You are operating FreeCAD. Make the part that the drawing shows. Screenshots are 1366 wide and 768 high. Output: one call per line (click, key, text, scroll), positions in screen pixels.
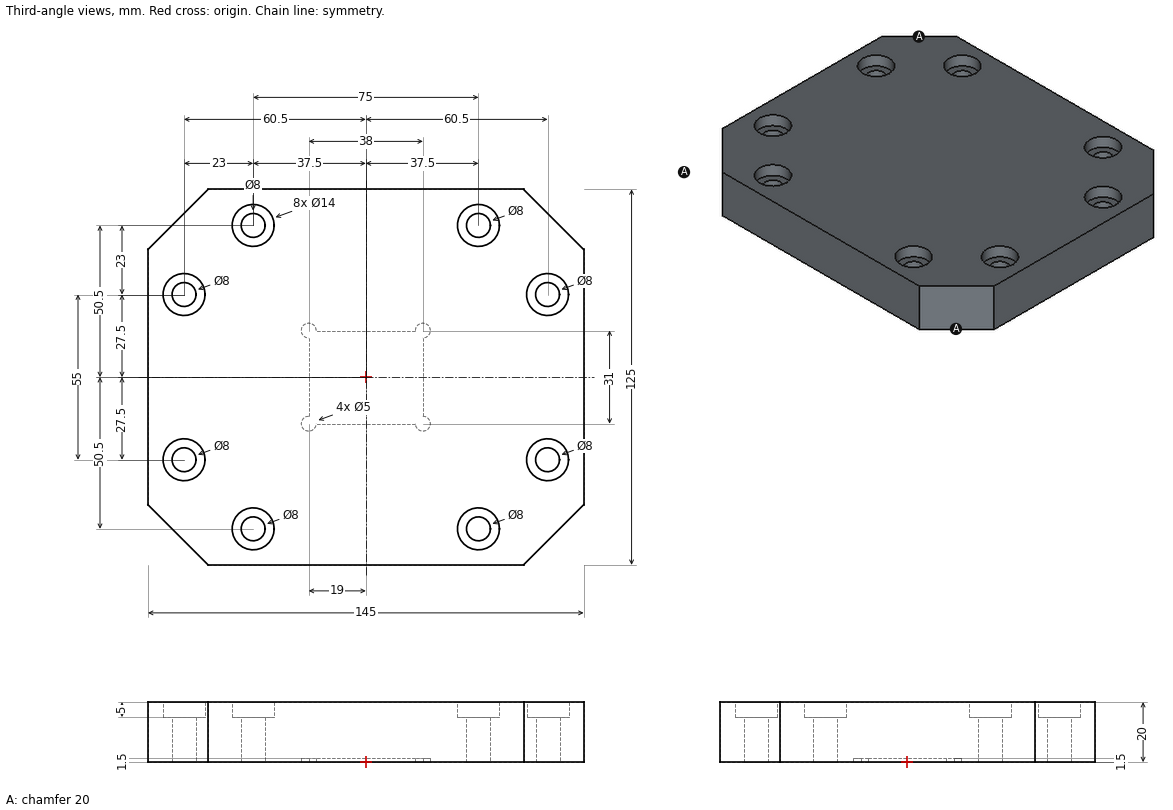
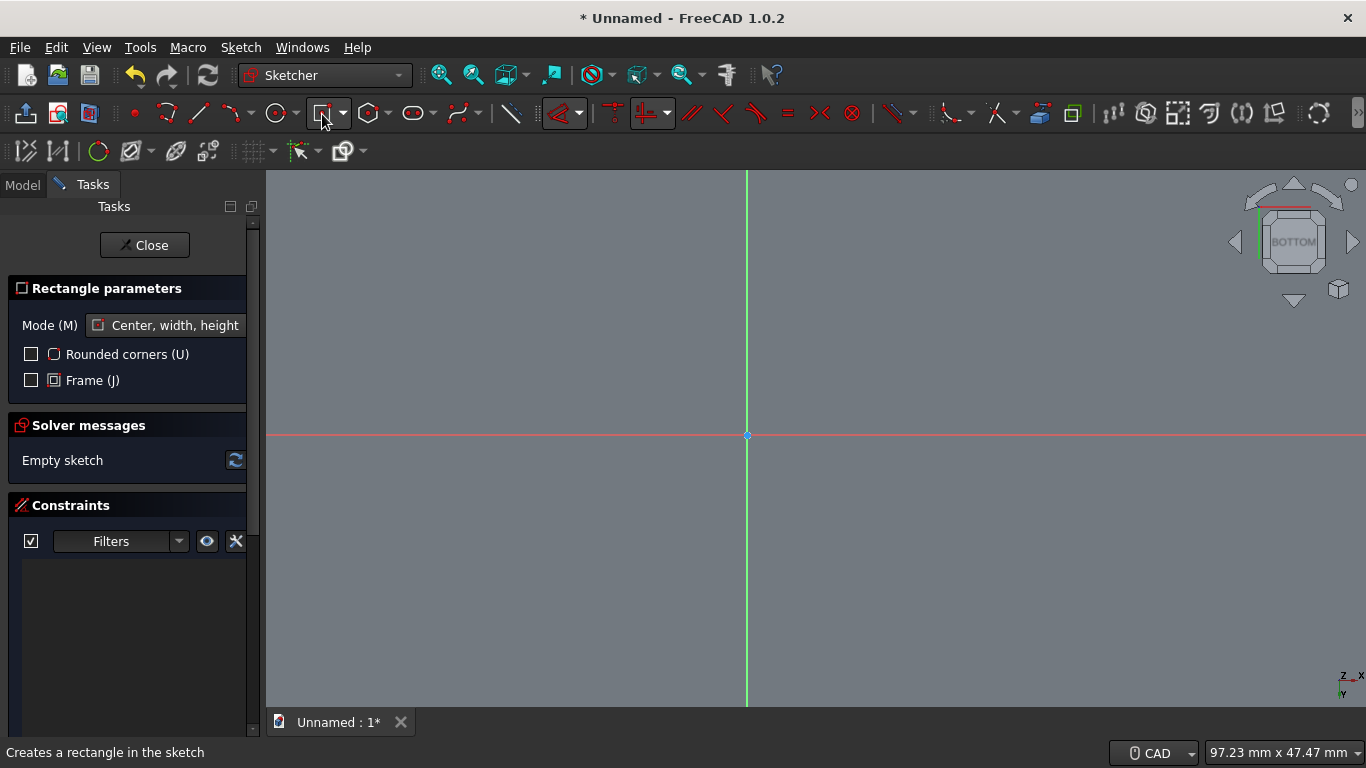
click(747, 435)
click(962, 260)
key(Escape)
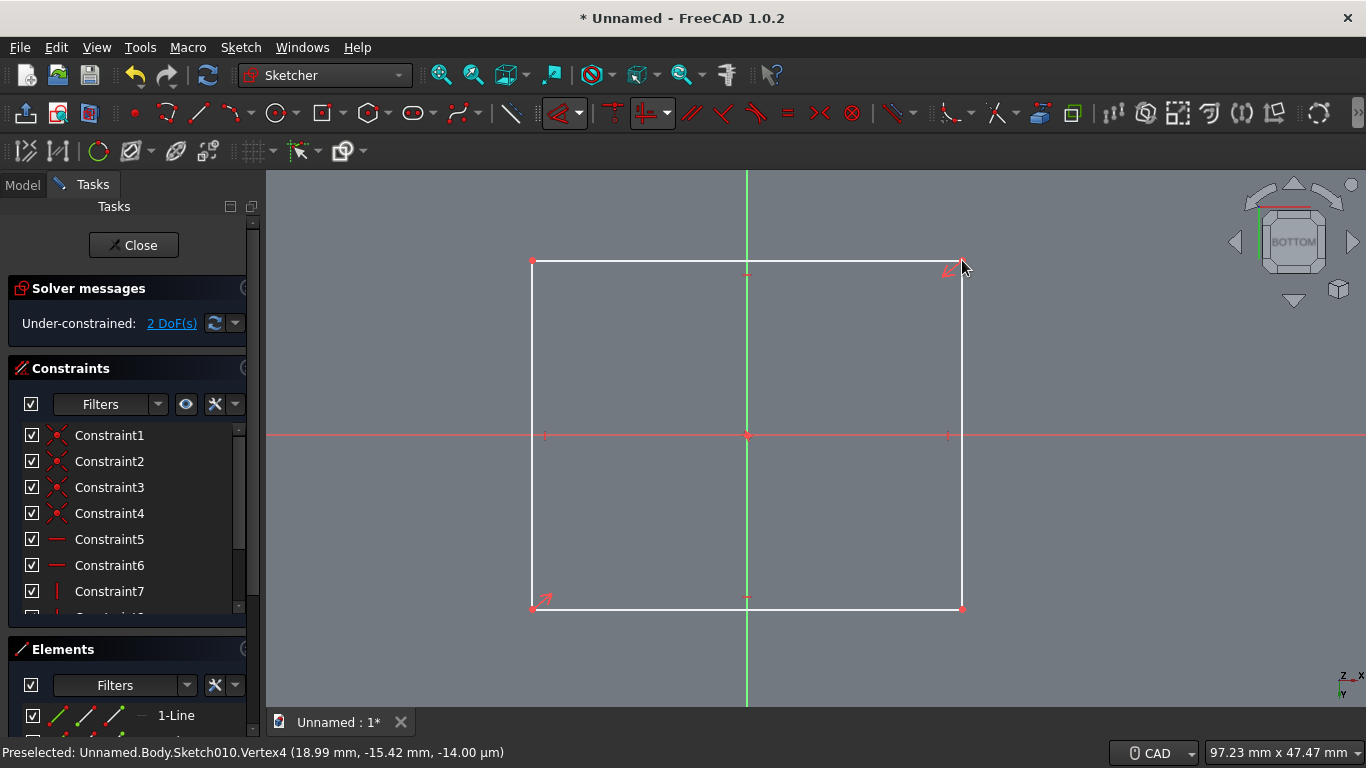
click(661, 610)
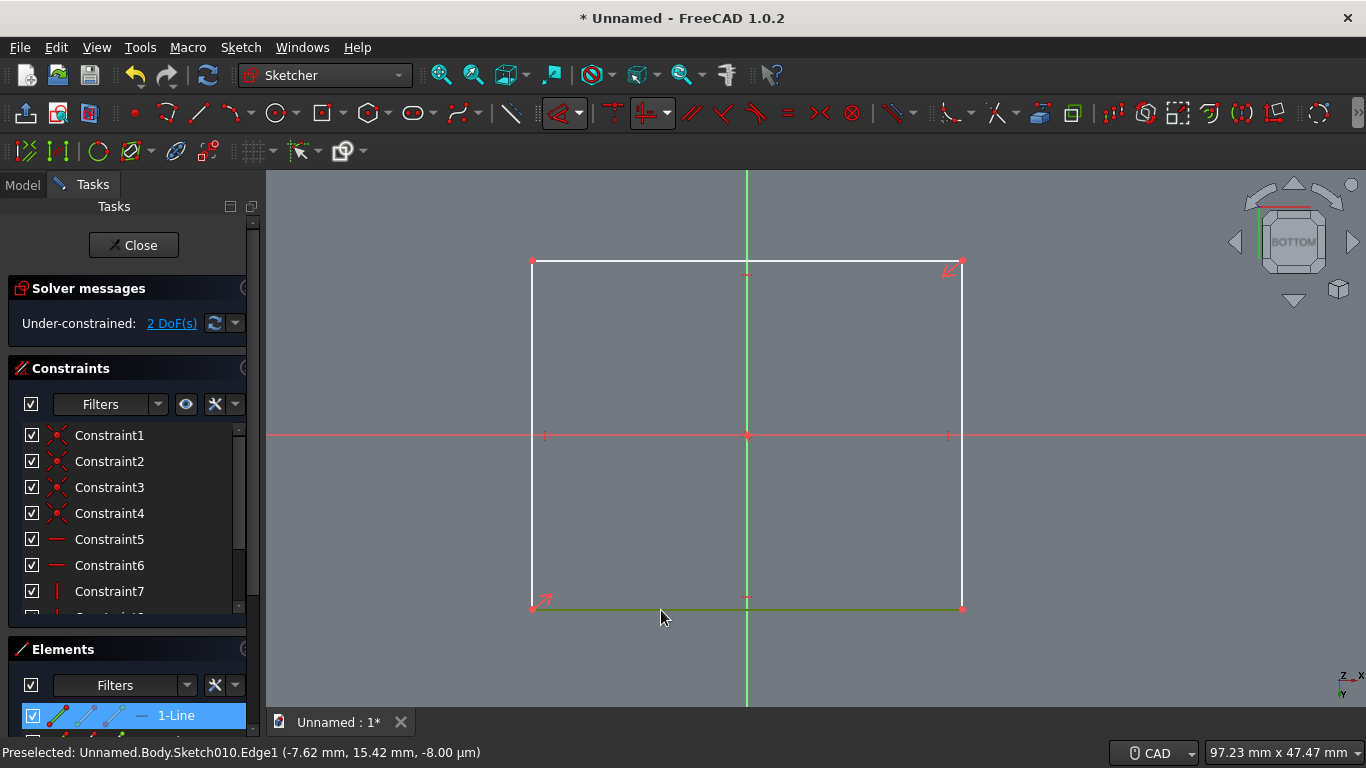
key(l)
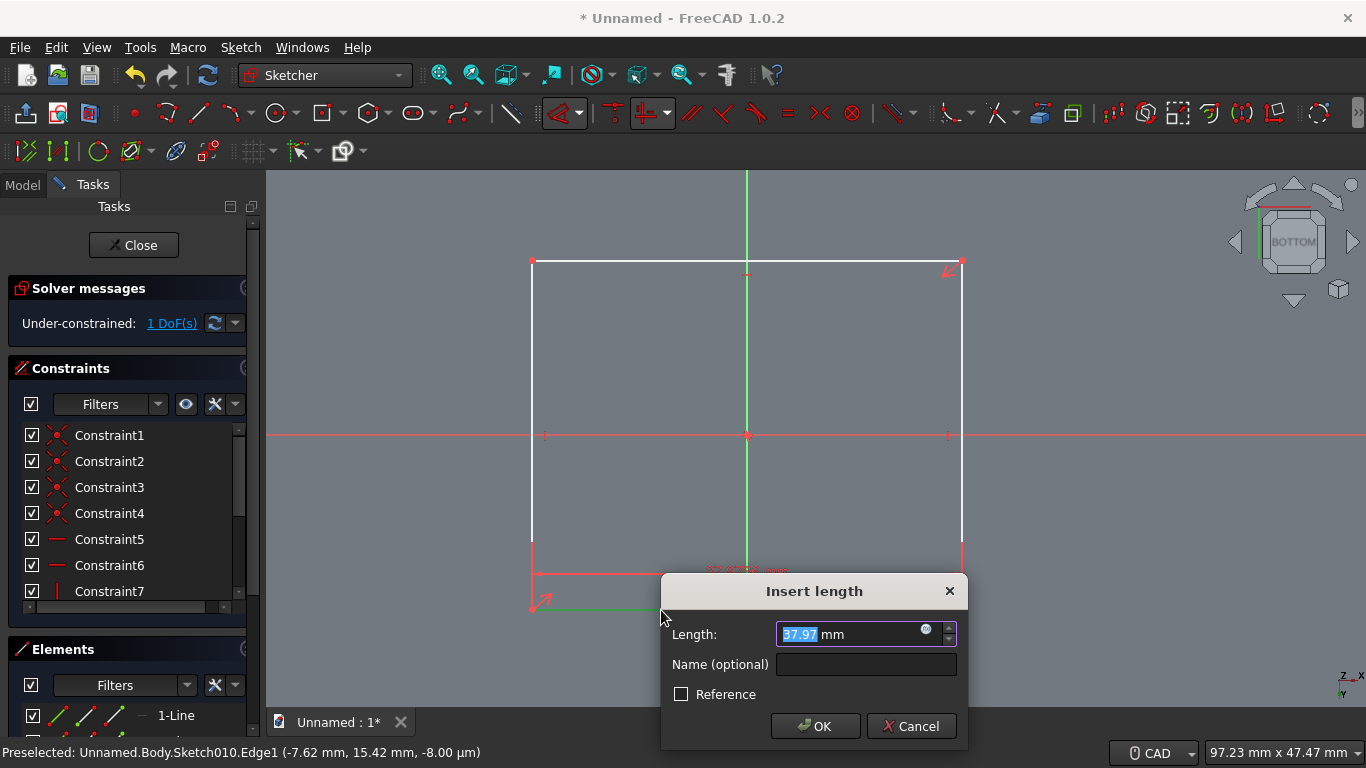
text(38)
key(Return)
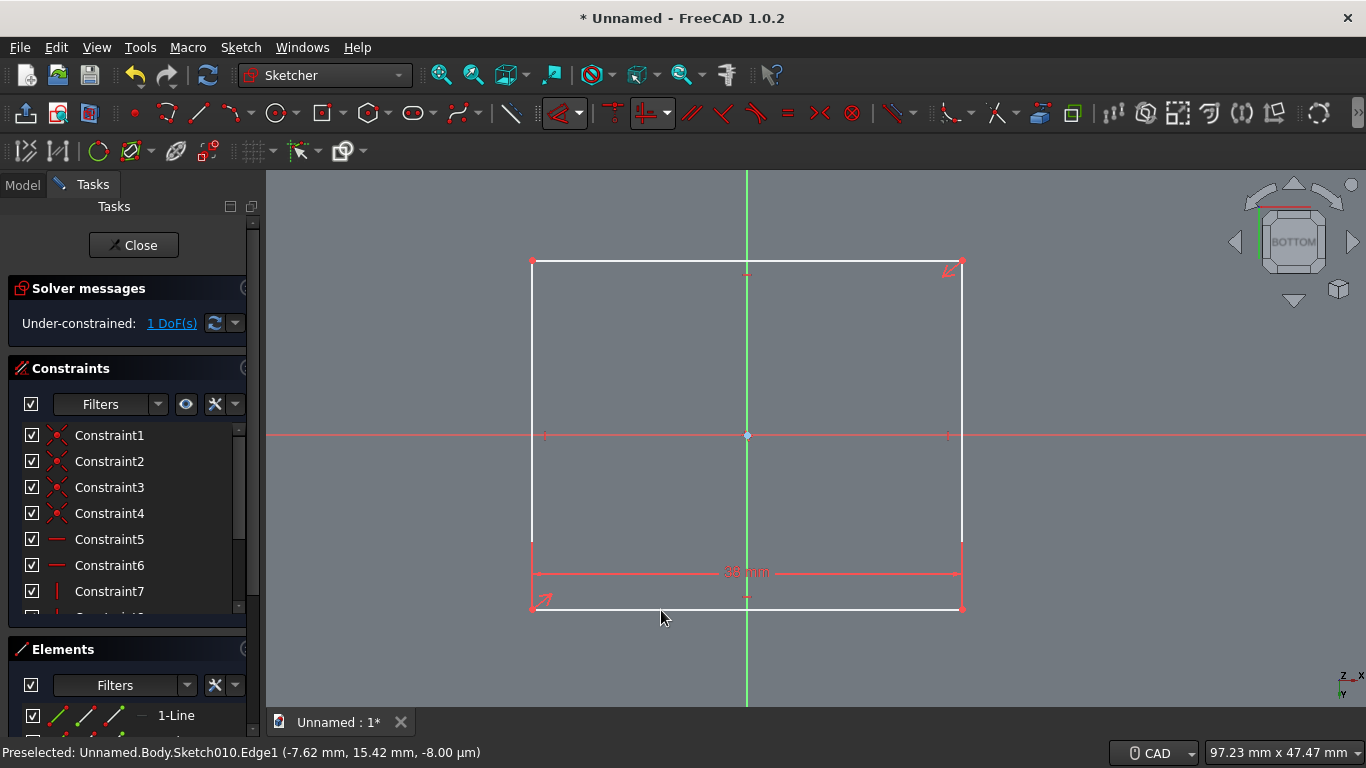
click(962, 505)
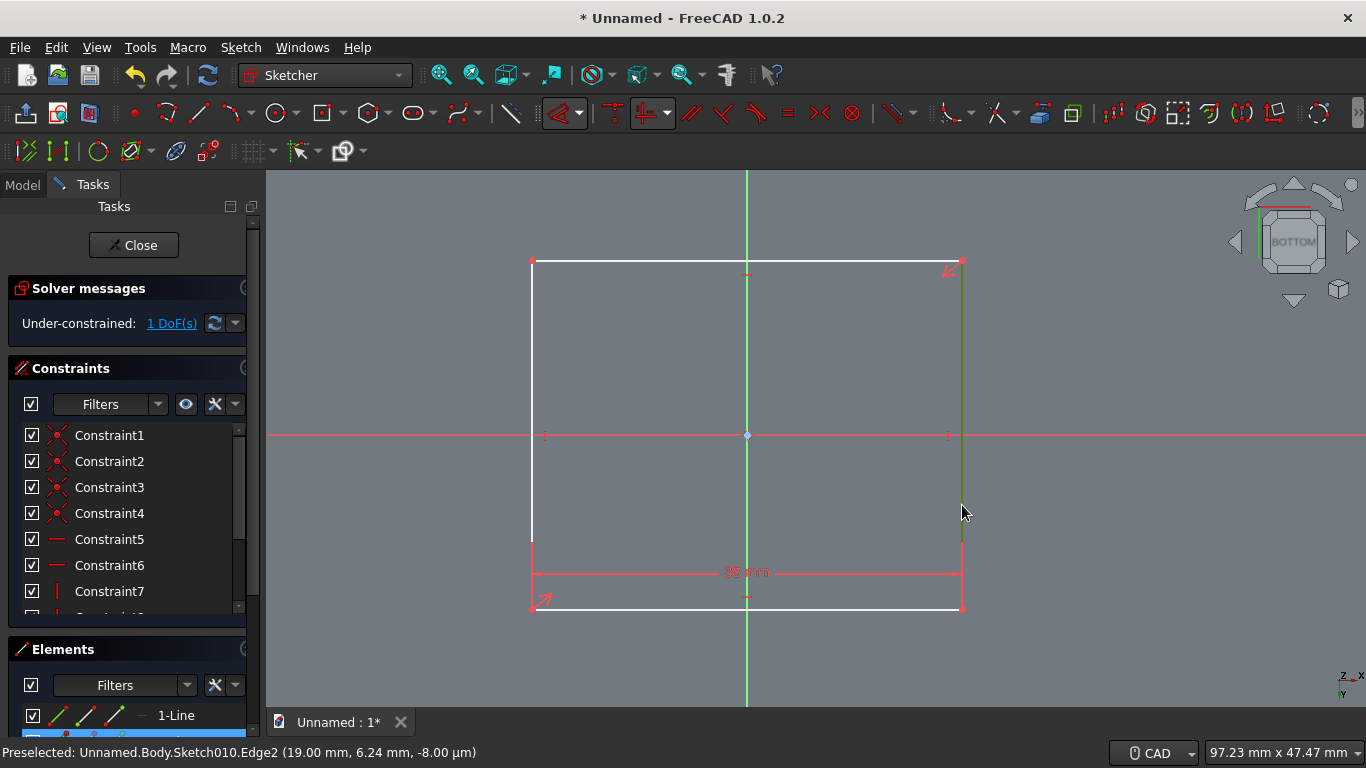
key(i)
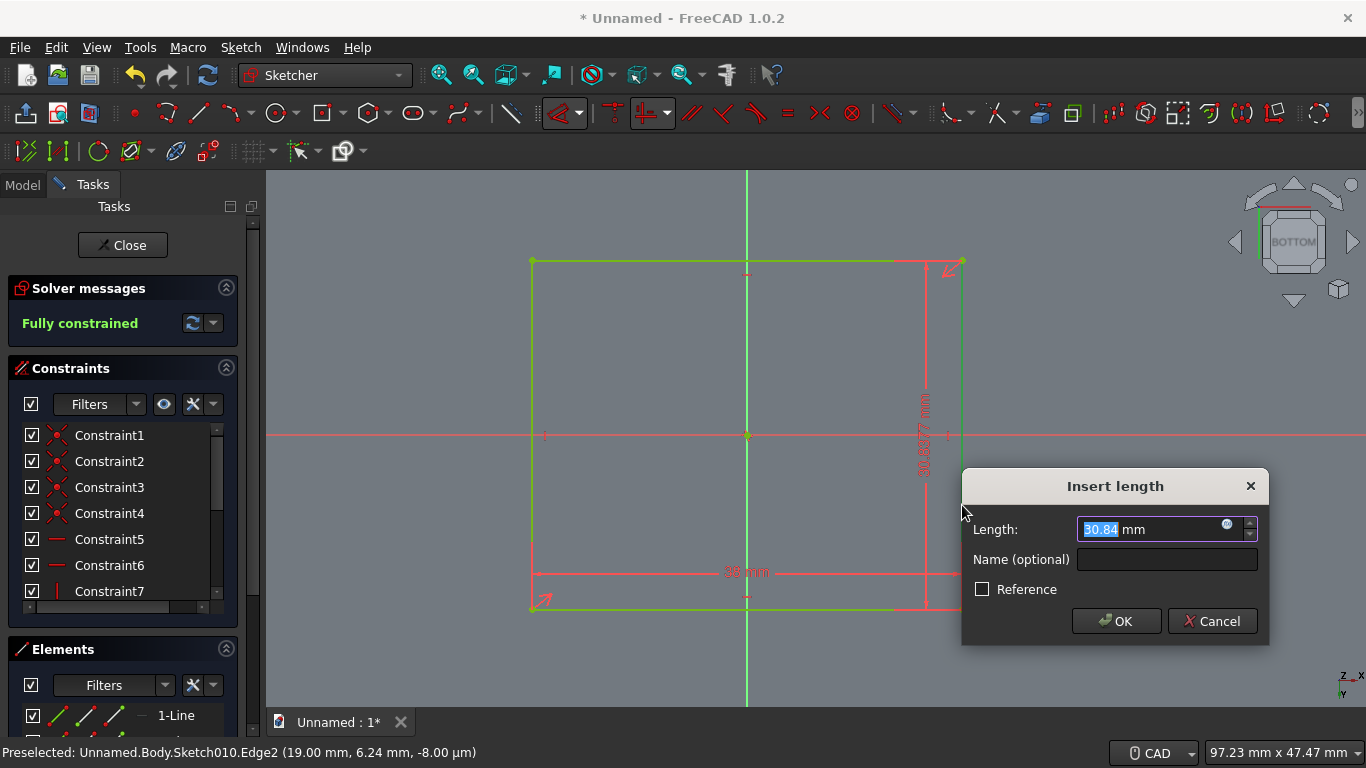
text(31)
key(Return)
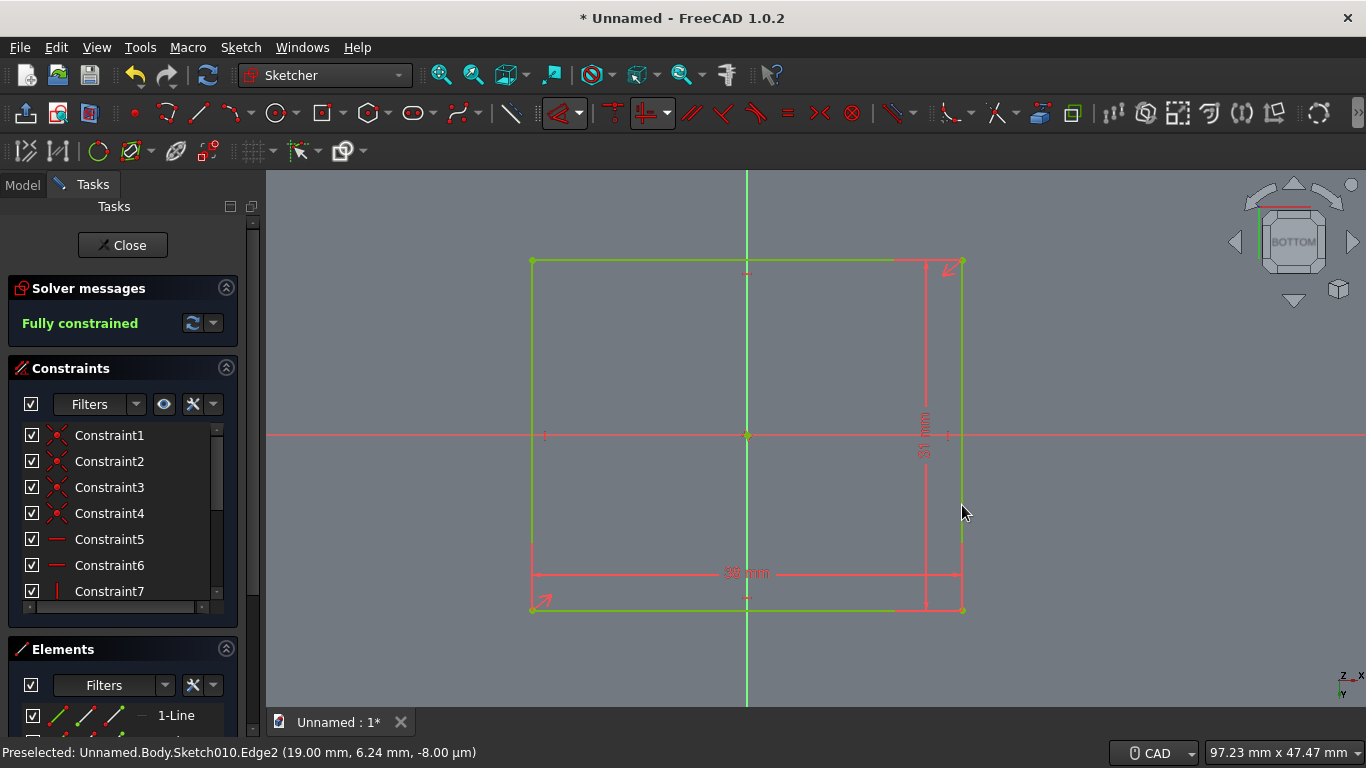
click(123, 245)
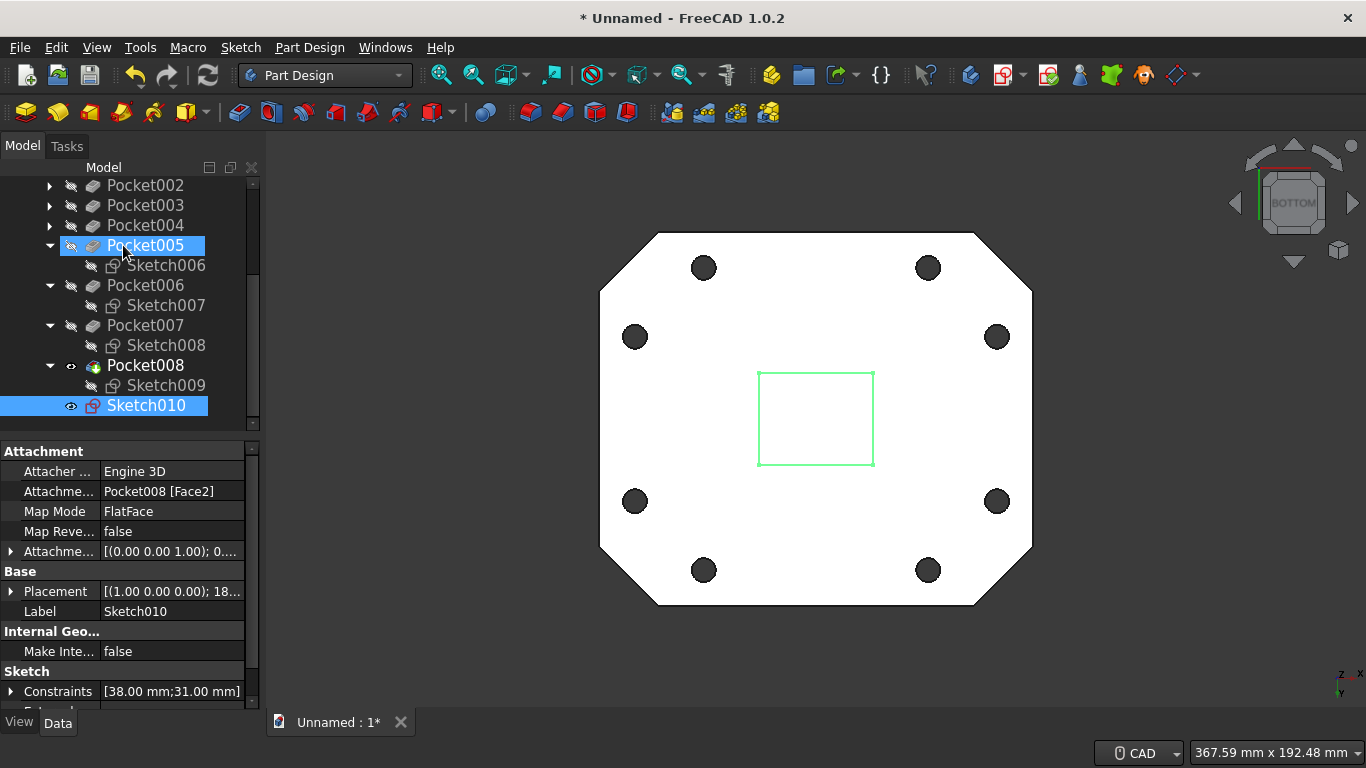
click(240, 112)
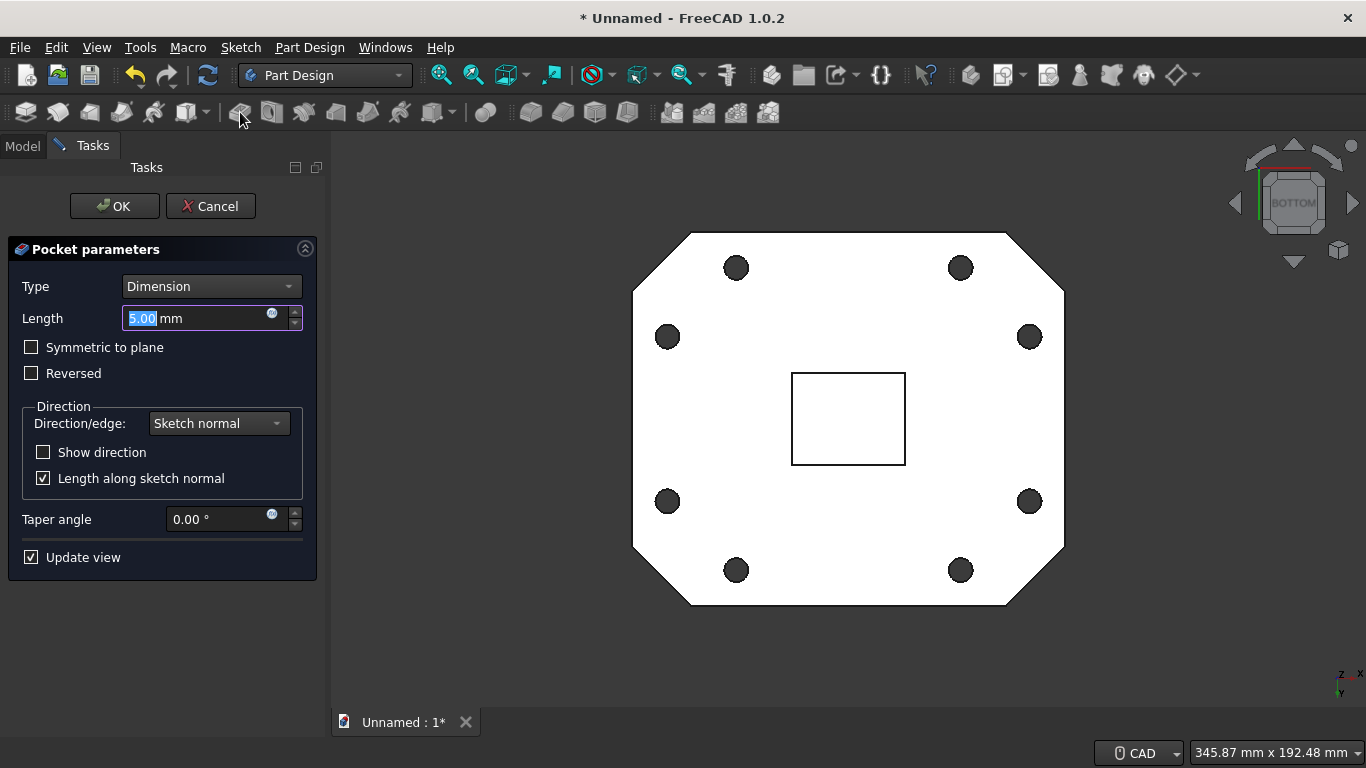
text(1.5)
key(Tab)